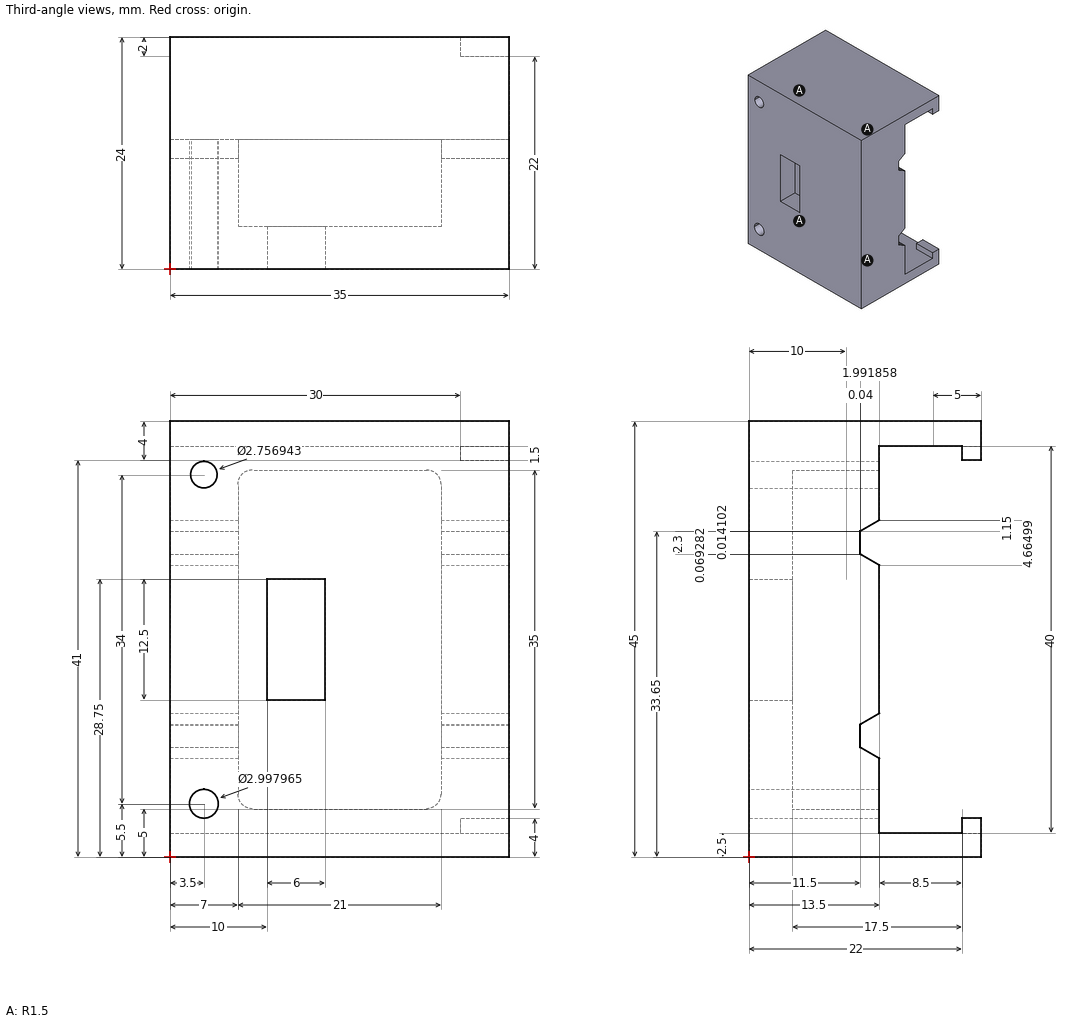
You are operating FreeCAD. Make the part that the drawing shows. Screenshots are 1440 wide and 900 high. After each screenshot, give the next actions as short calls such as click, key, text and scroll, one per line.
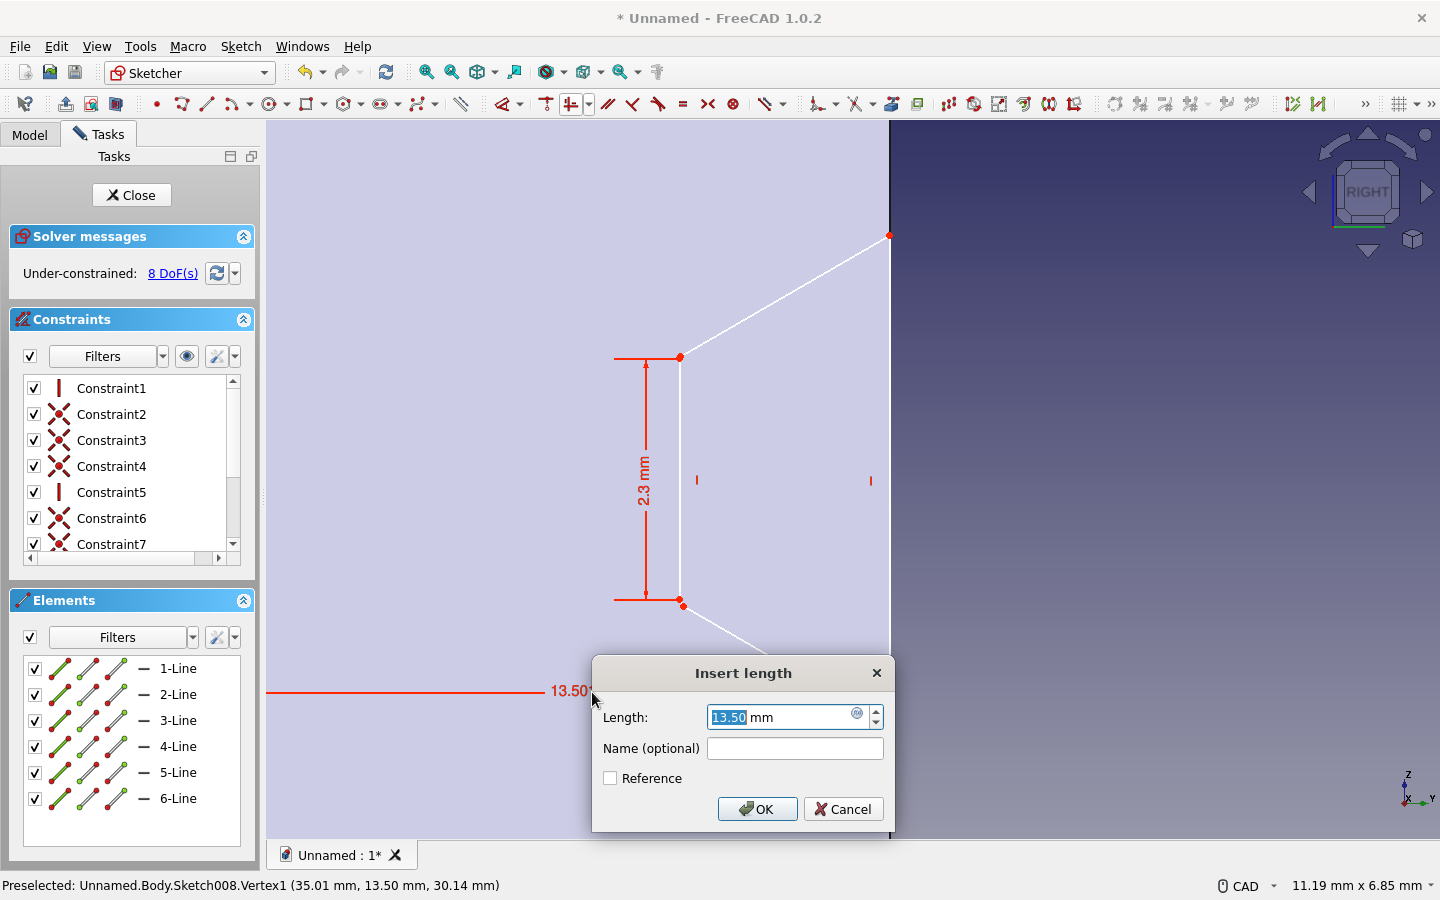
text(13.5)
key(Return)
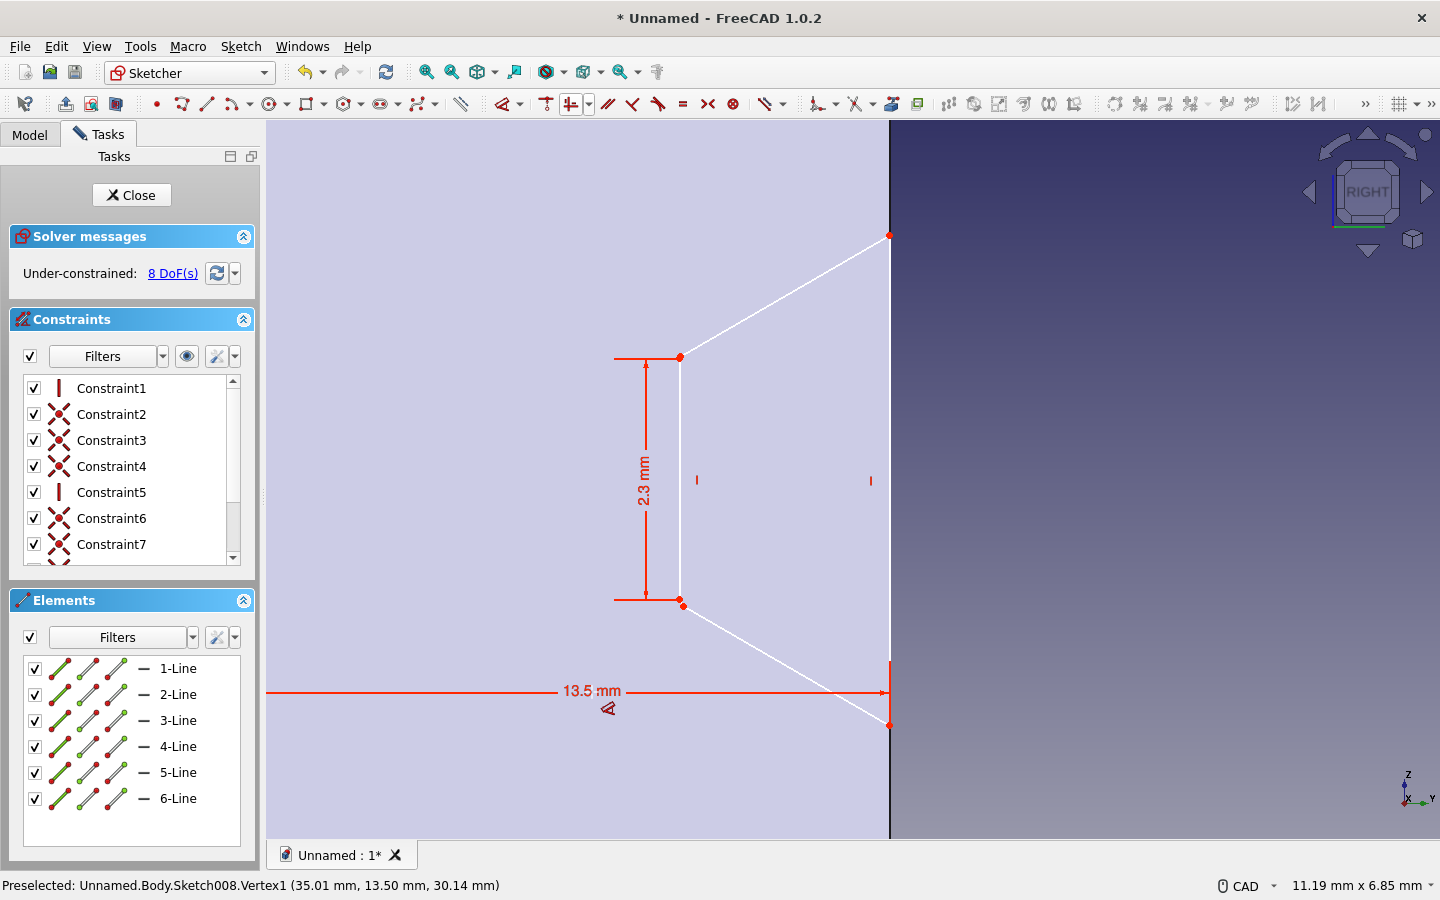
scroll(680, 359, up, 9)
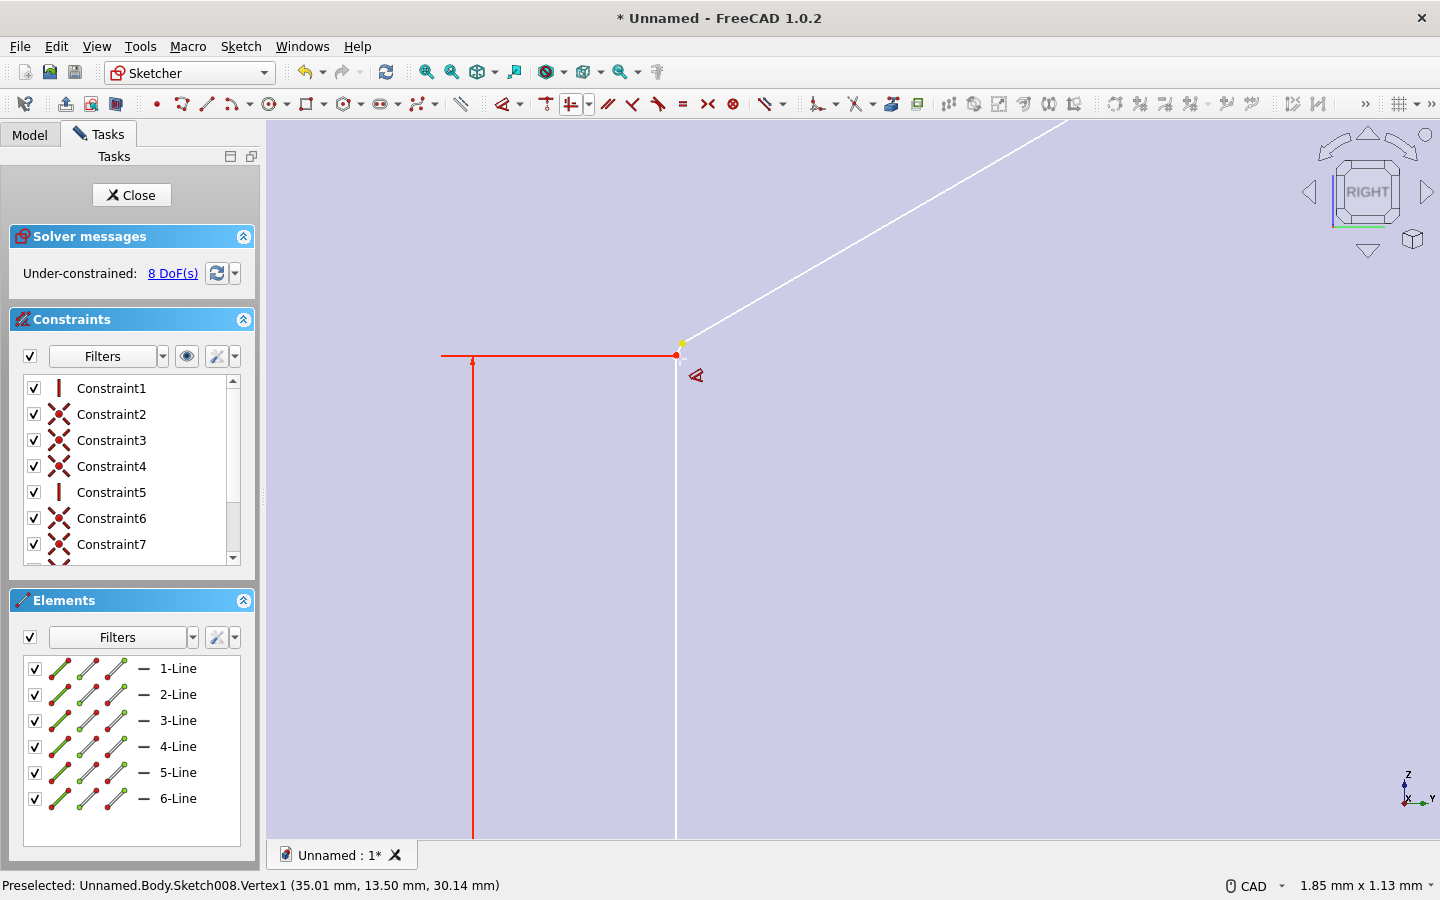
click(676, 356)
click(485, 322)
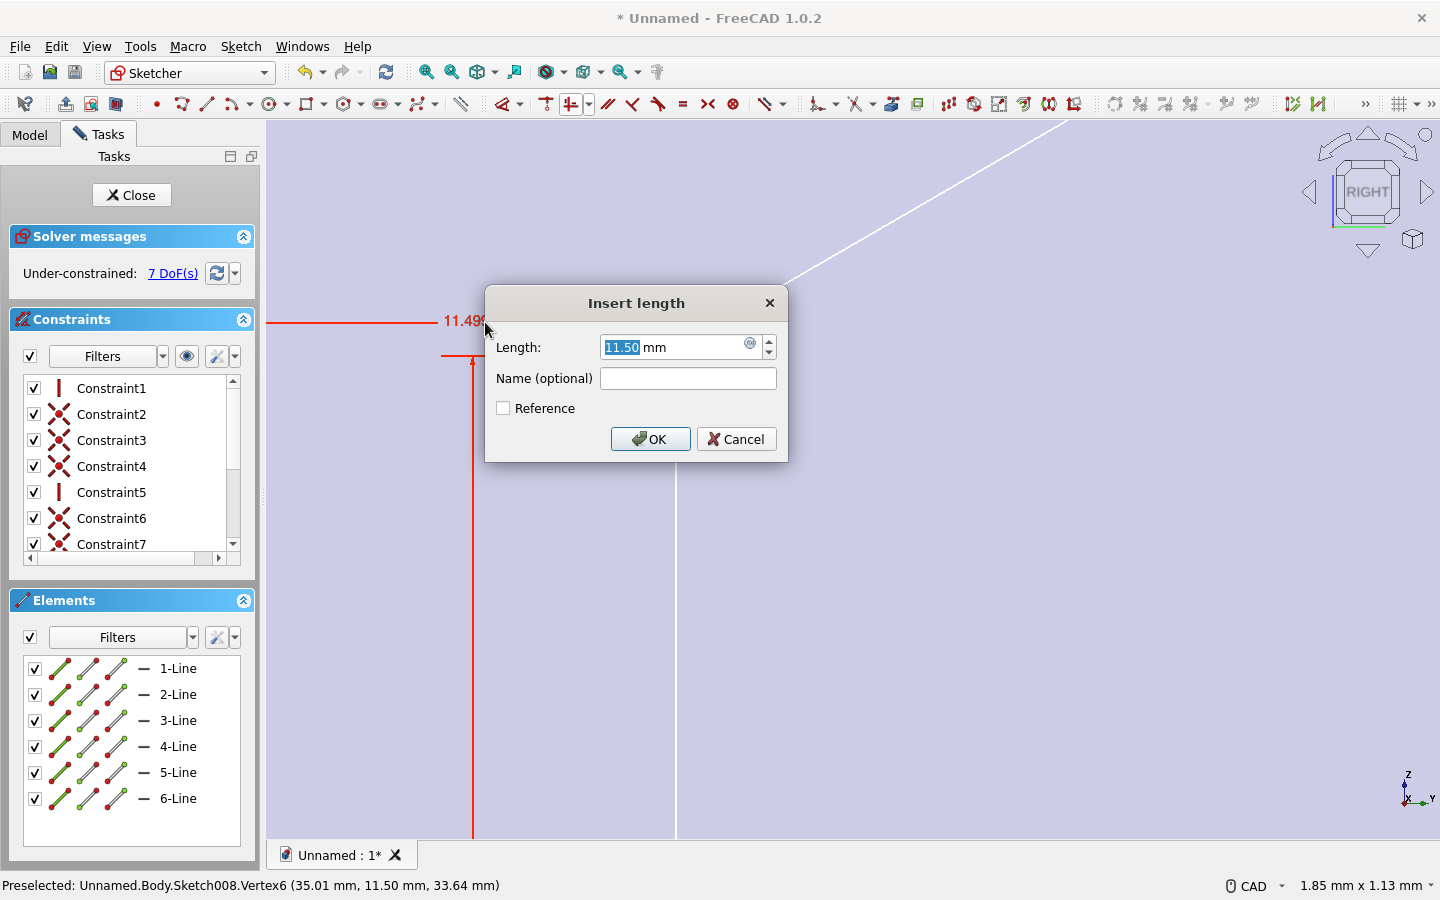
text(11.5)
key(Return)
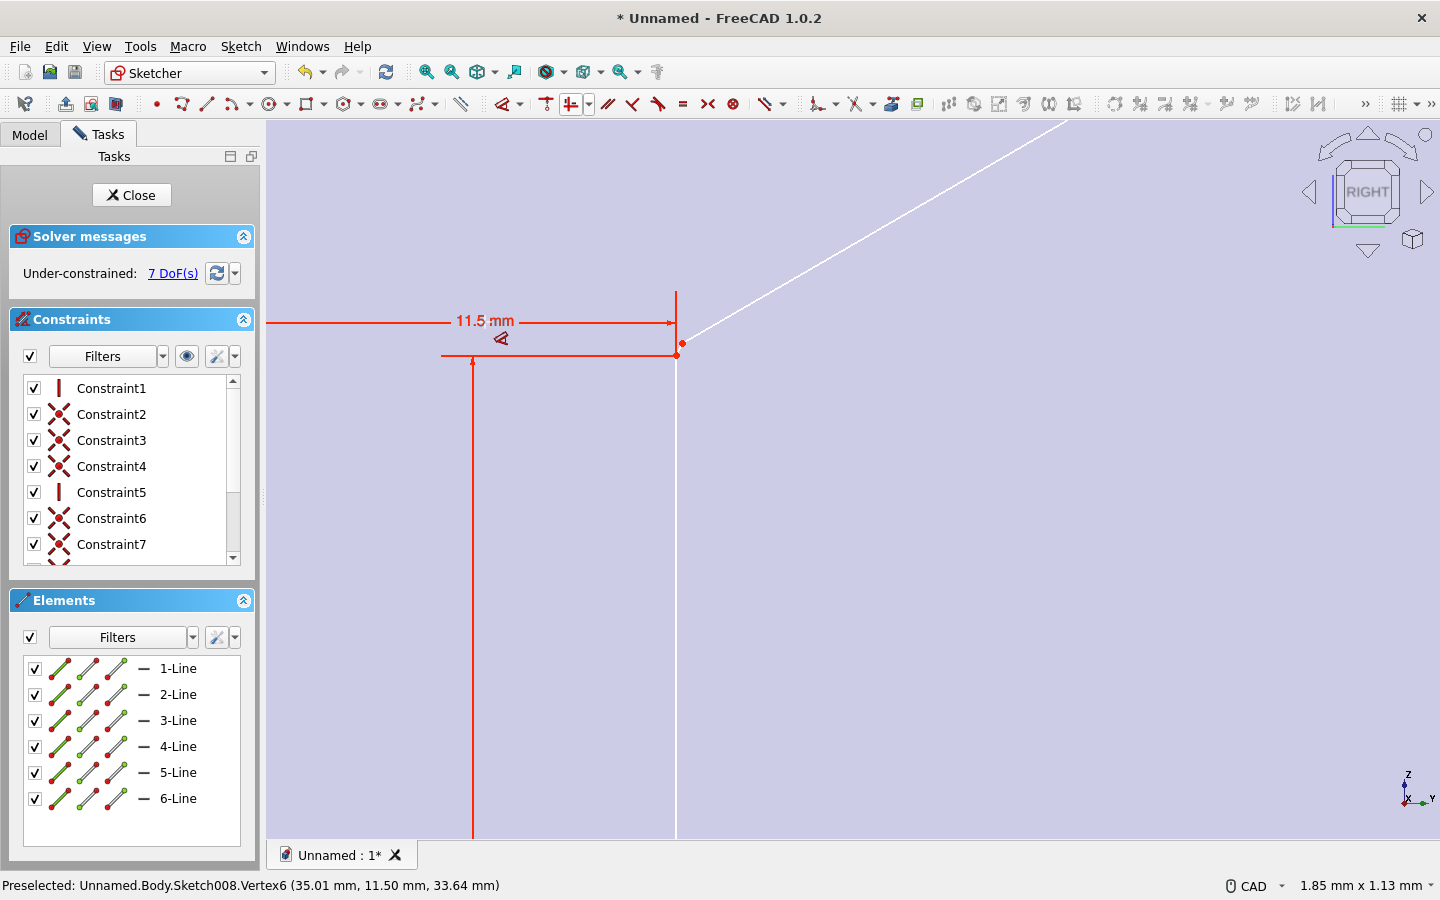
scroll(680, 359, down, 9)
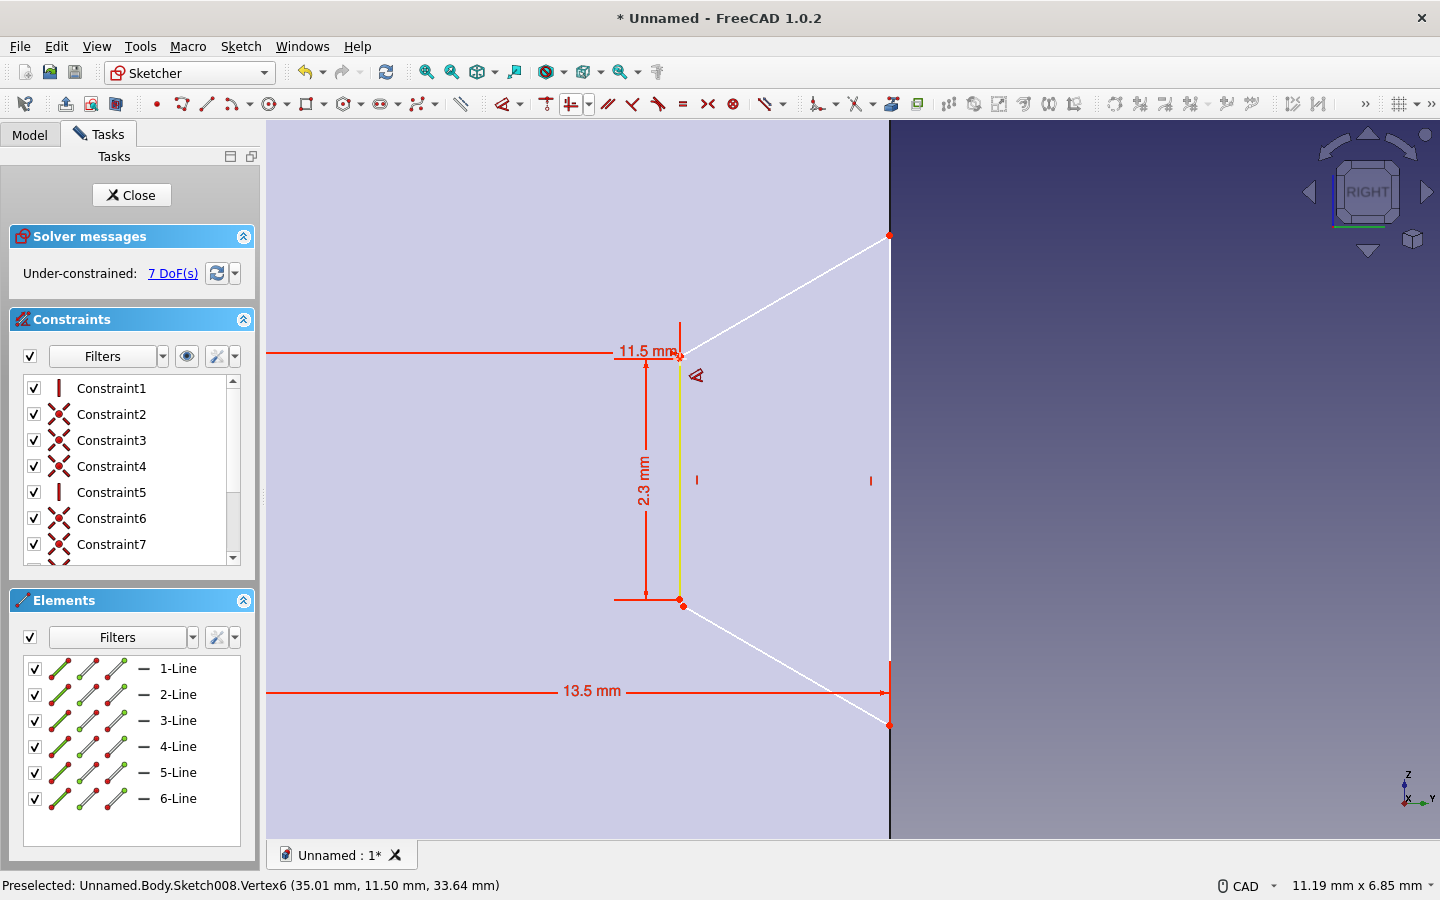
click(722, 333)
click(924, 296)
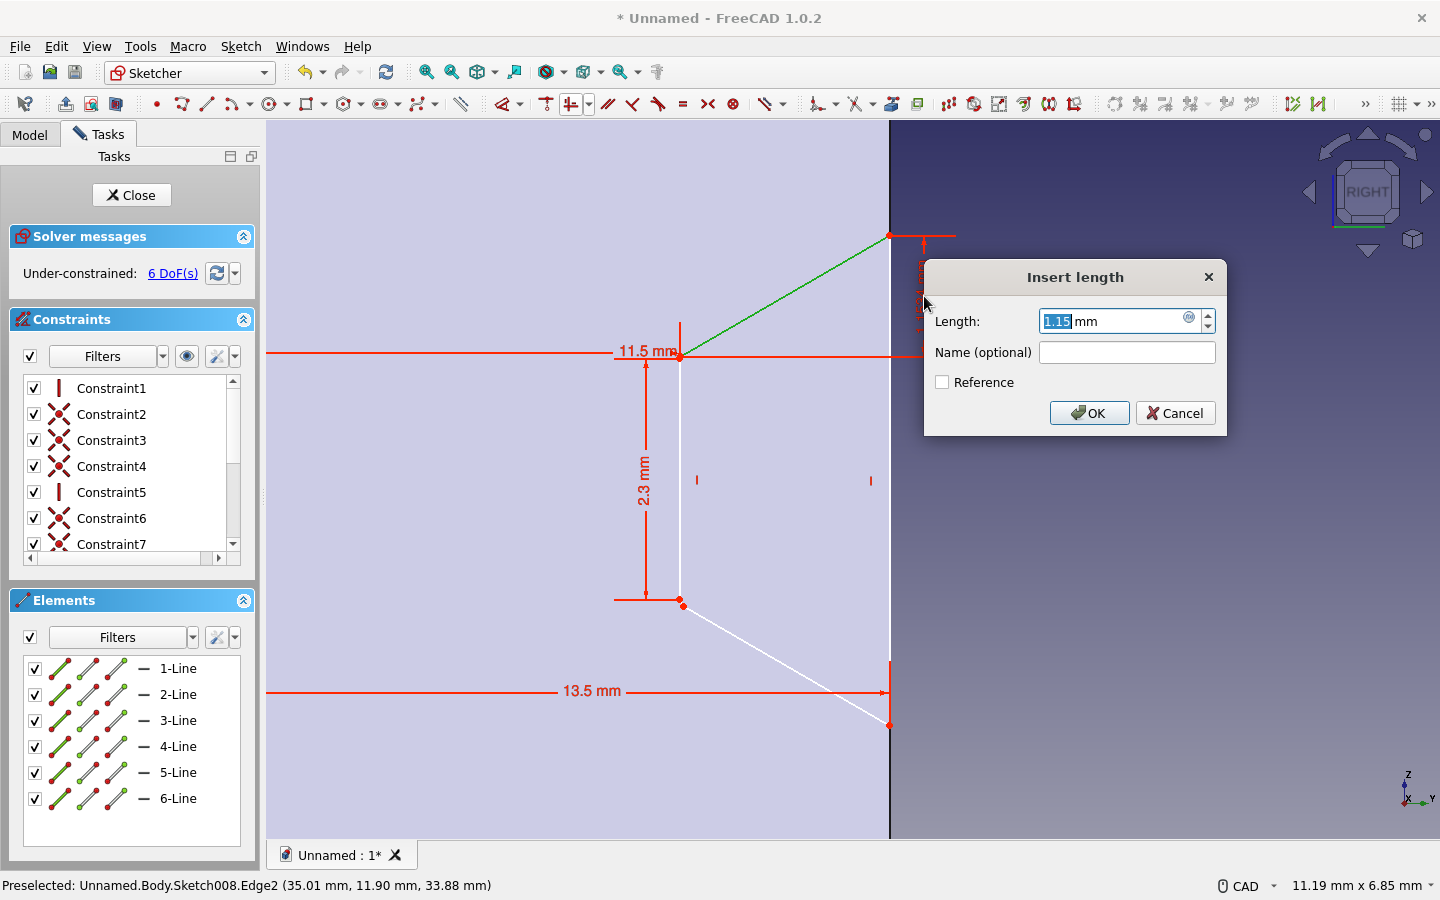
text(1.15)
key(Return)